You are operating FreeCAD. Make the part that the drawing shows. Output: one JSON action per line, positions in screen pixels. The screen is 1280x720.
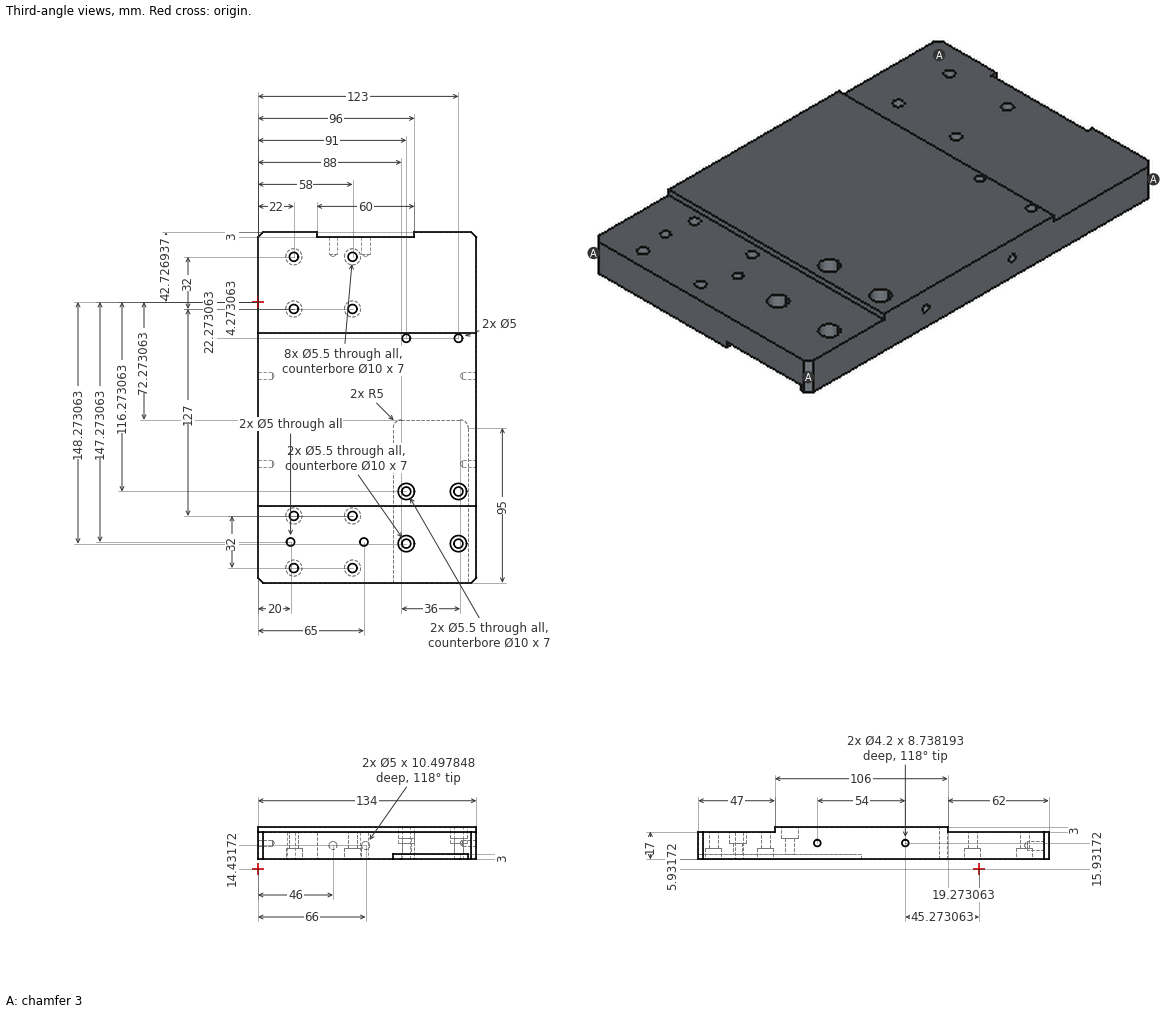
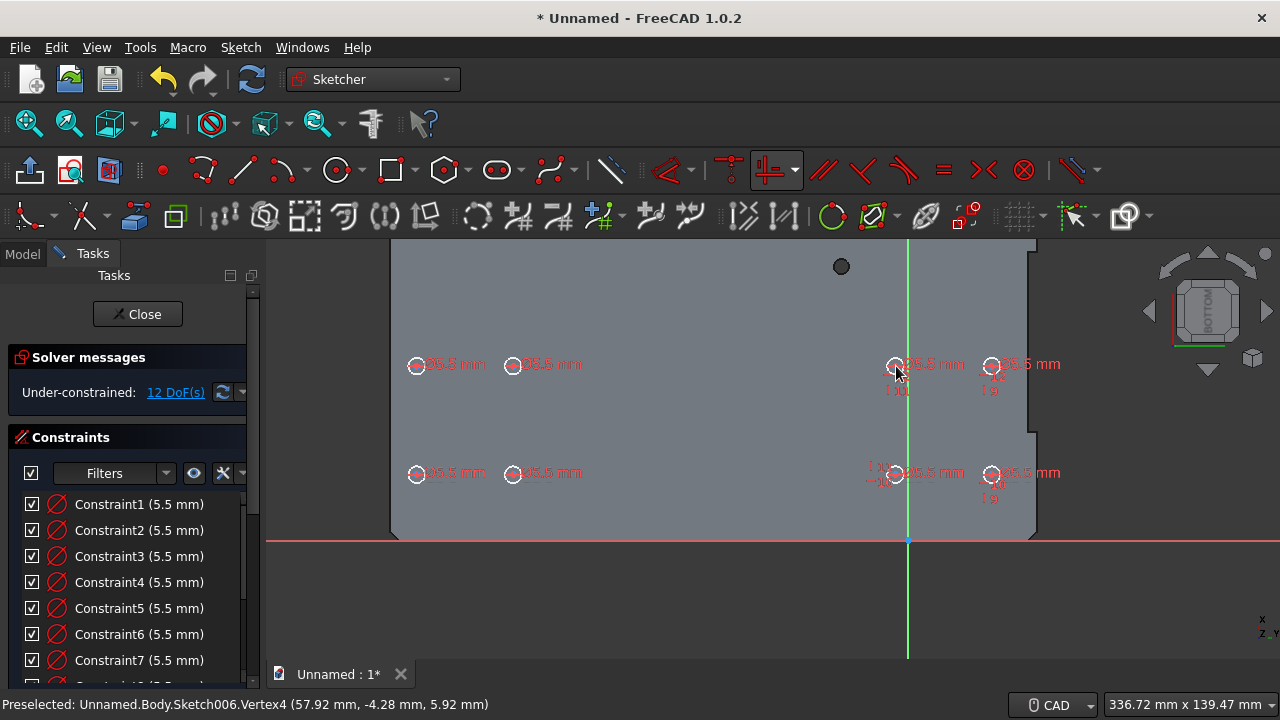
{"action": "left_click", "coordinate": [896, 366]}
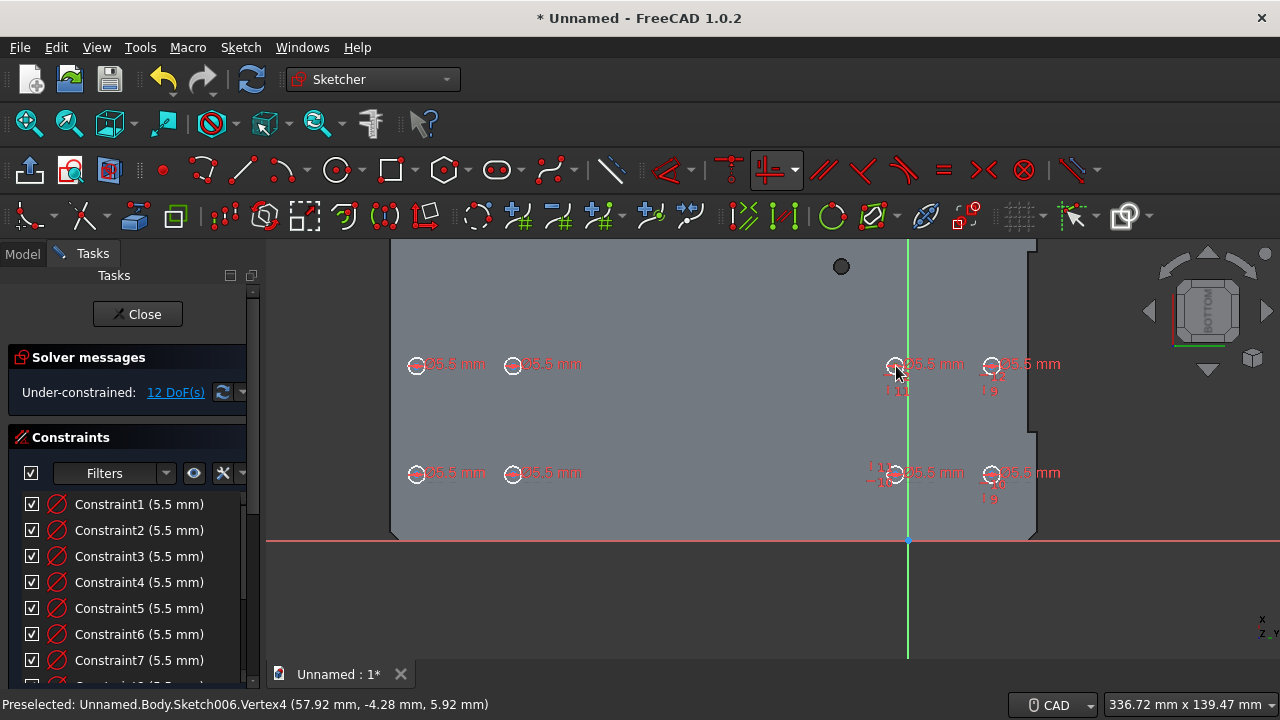
{"action": "left_click", "coordinate": [513, 366]}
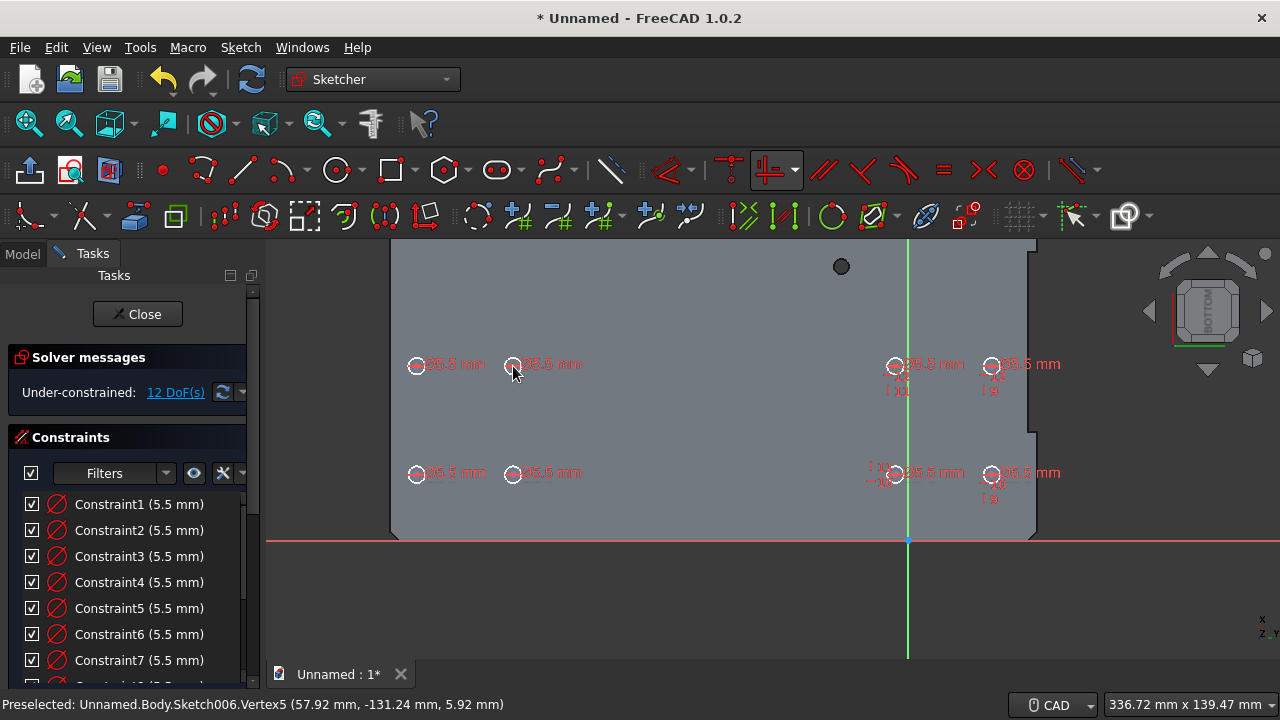
{"action": "key", "text": "h"}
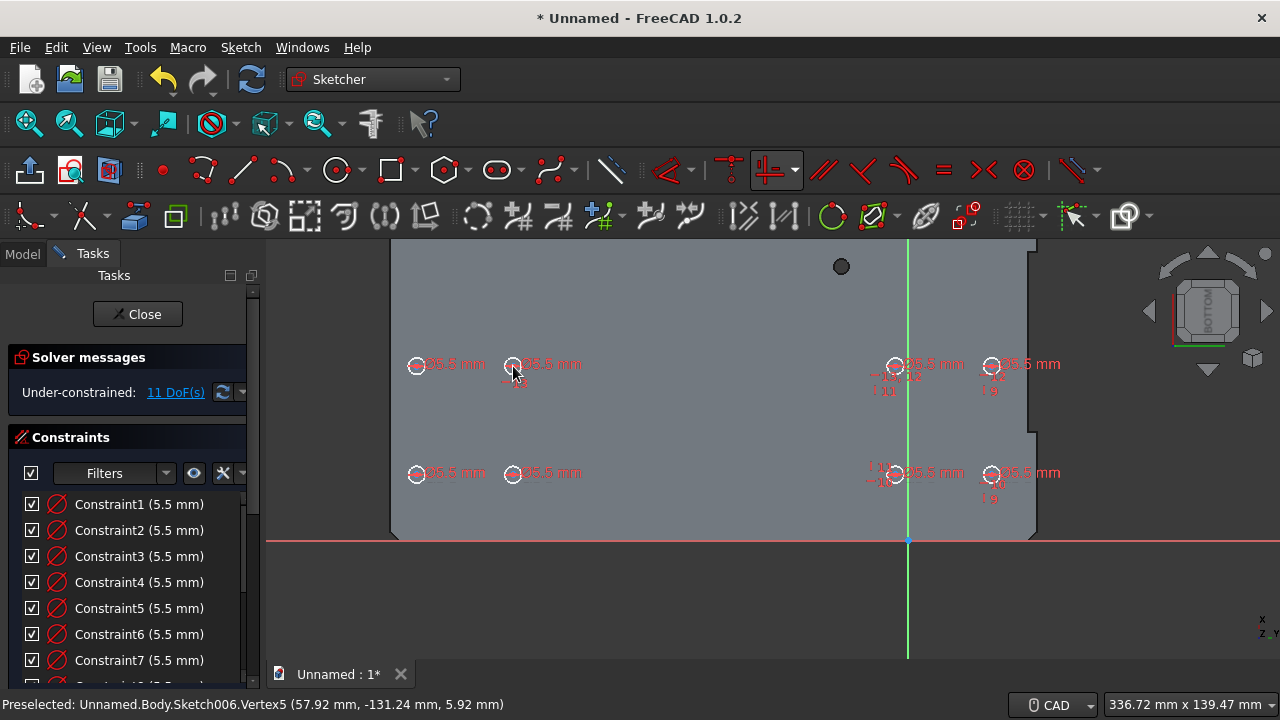
{"action": "left_click", "coordinate": [513, 366]}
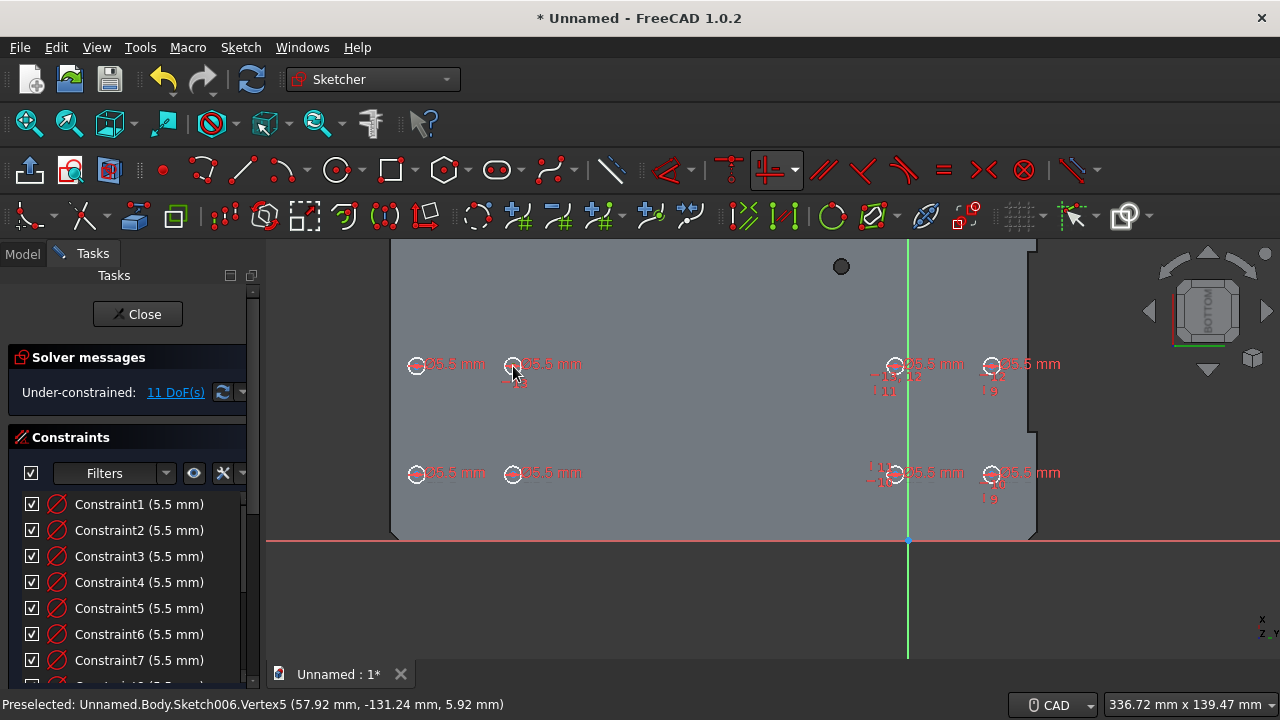
{"action": "left_click", "coordinate": [417, 366]}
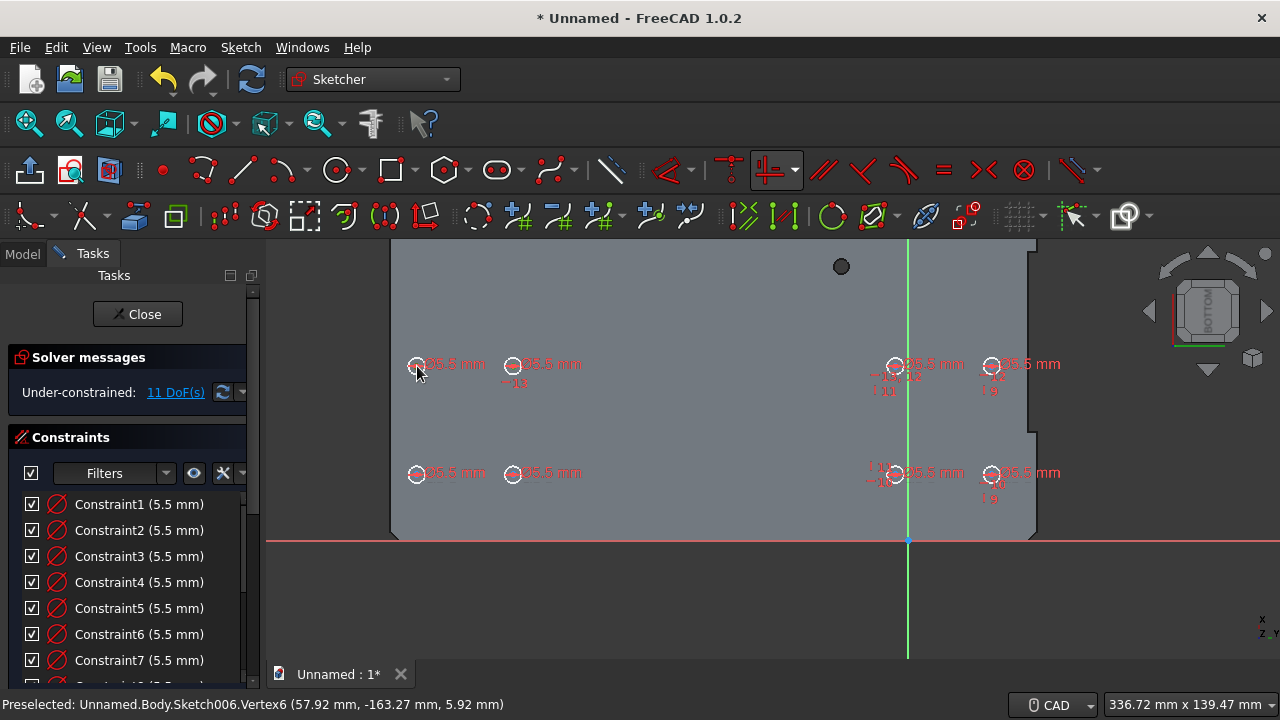
{"action": "key", "text": "h"}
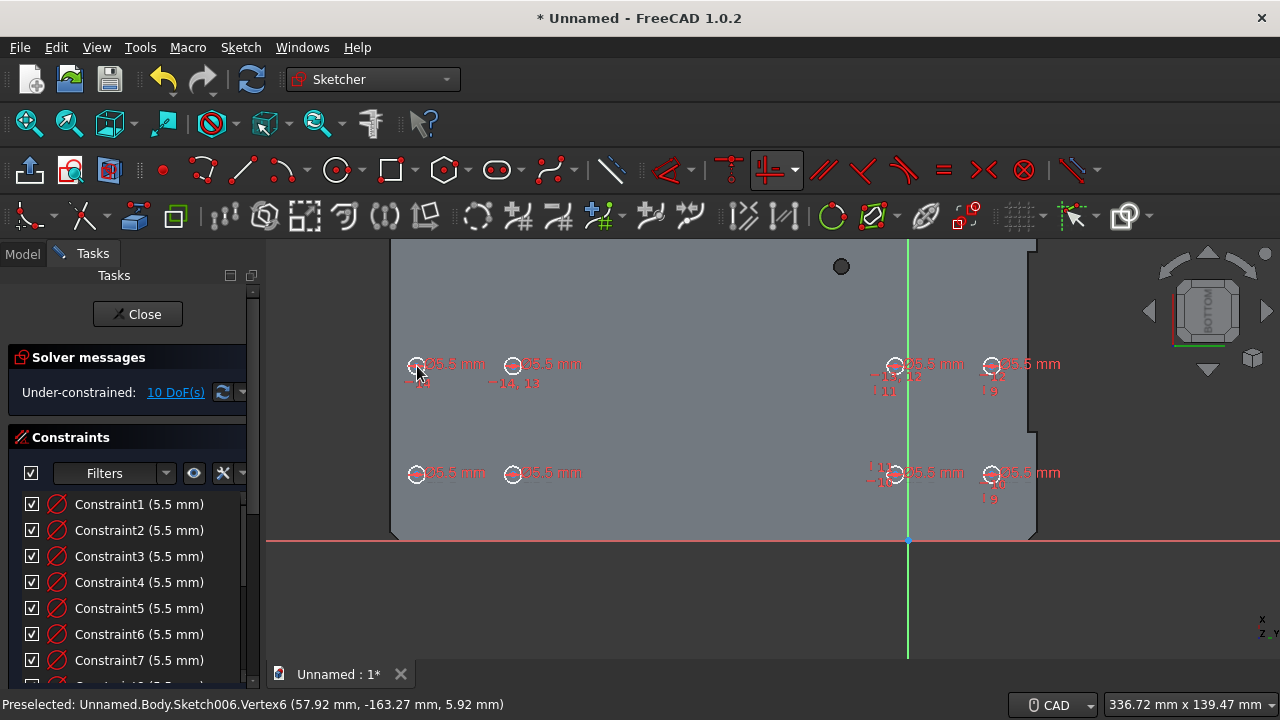
{"action": "left_click", "coordinate": [417, 366]}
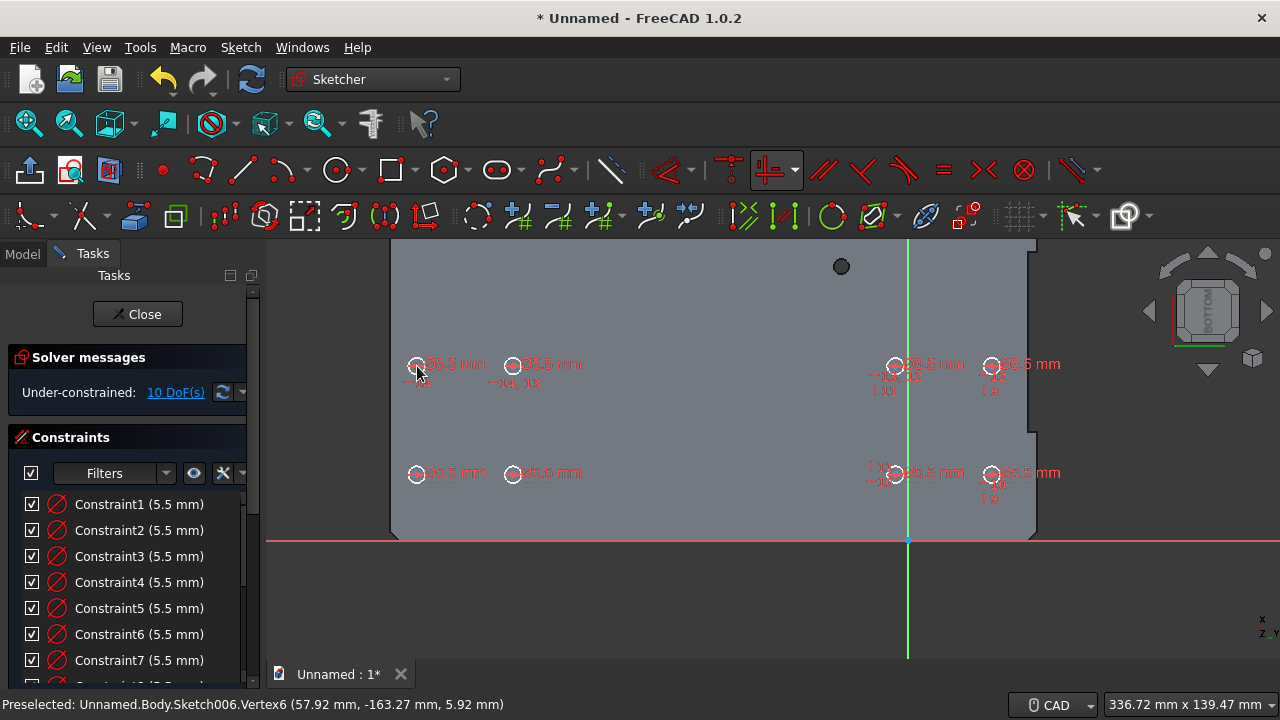
{"action": "left_click", "coordinate": [417, 475]}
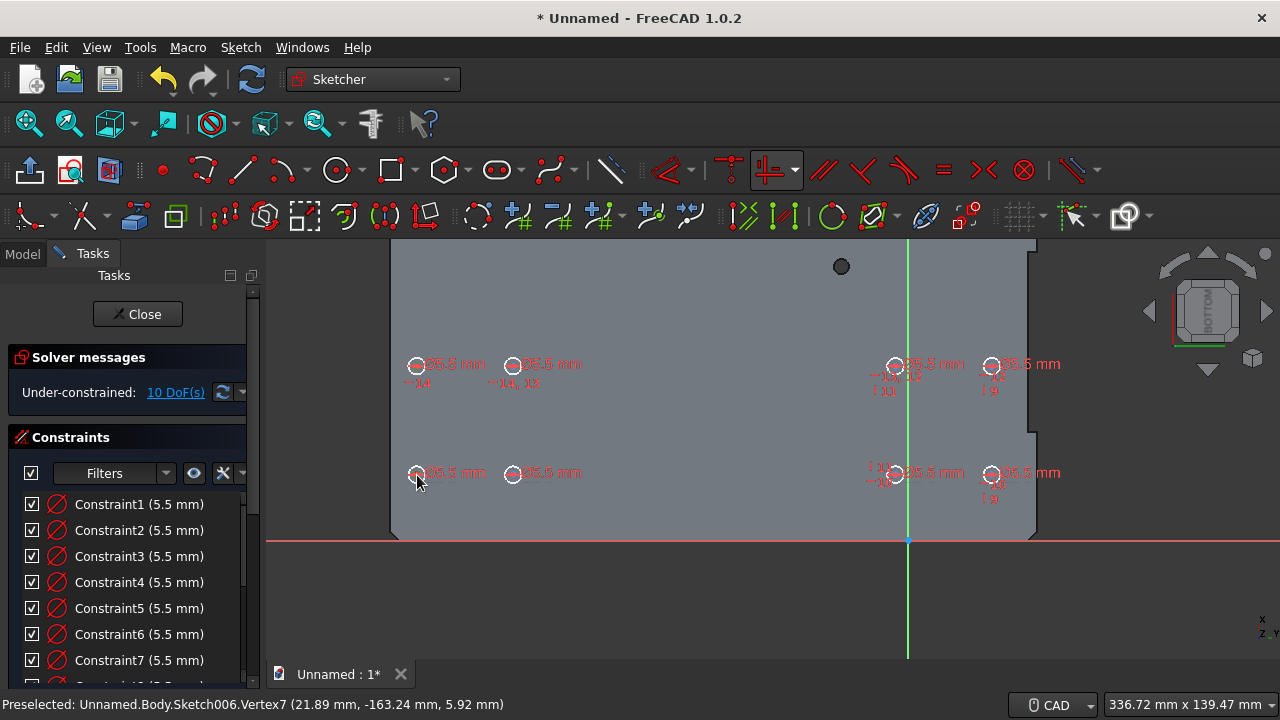
{"action": "left_click", "coordinate": [798, 170]}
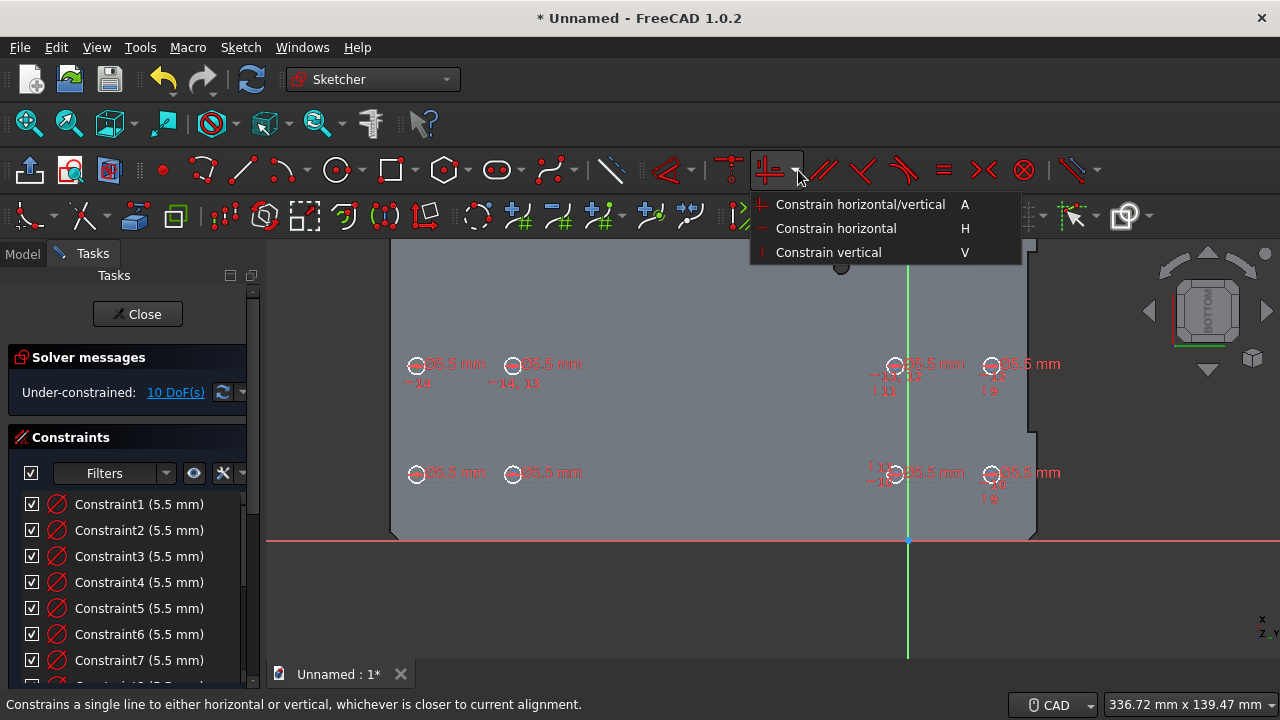
{"action": "left_click", "coordinate": [886, 252]}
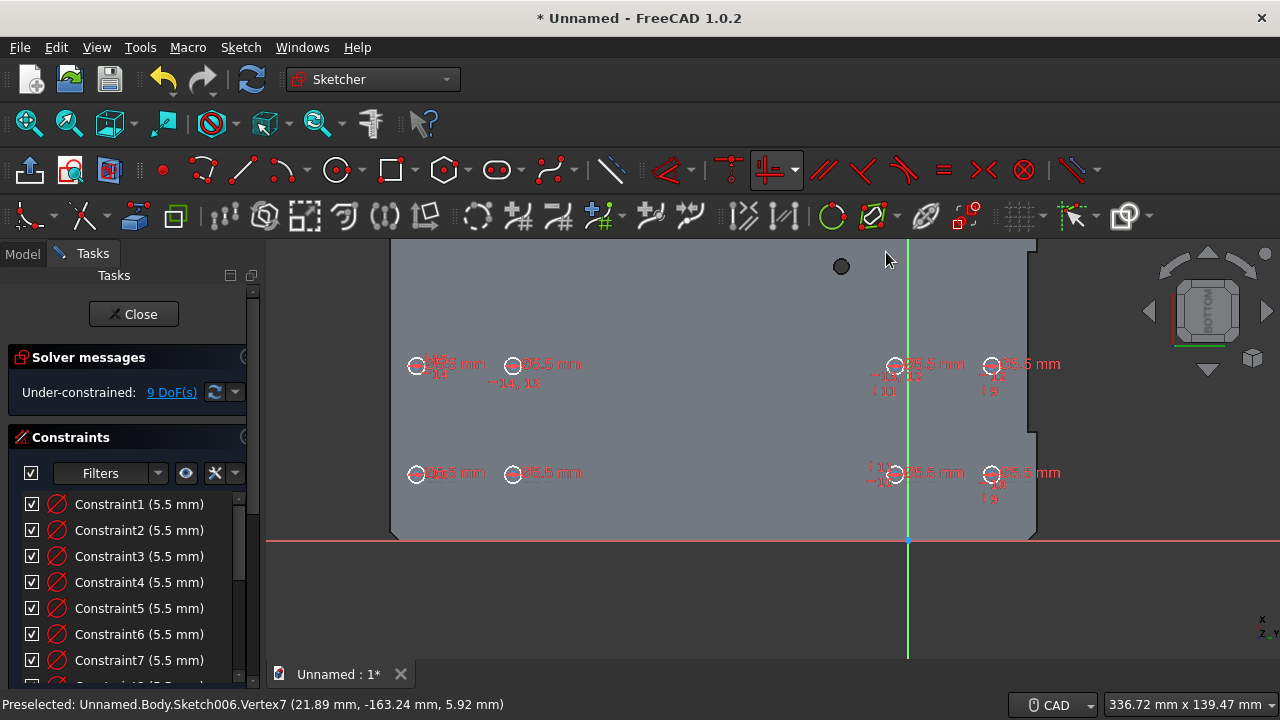
{"action": "left_click", "coordinate": [896, 475]}